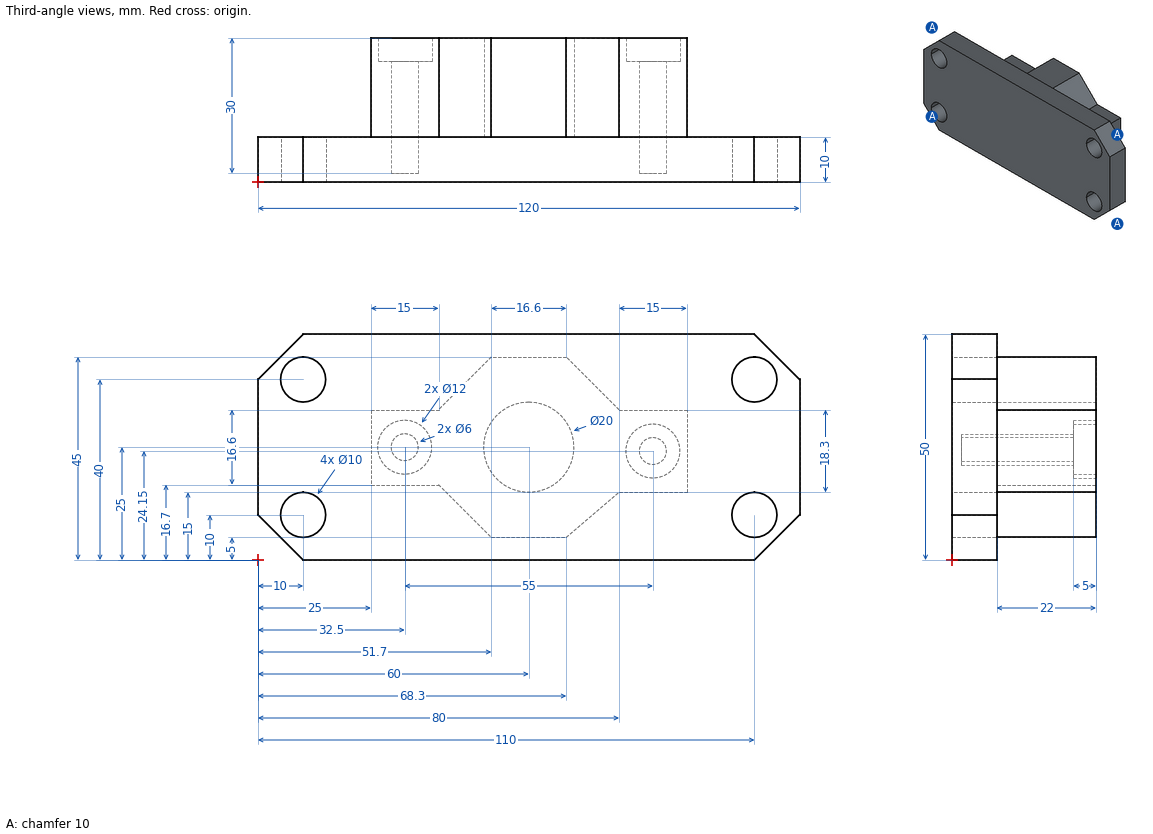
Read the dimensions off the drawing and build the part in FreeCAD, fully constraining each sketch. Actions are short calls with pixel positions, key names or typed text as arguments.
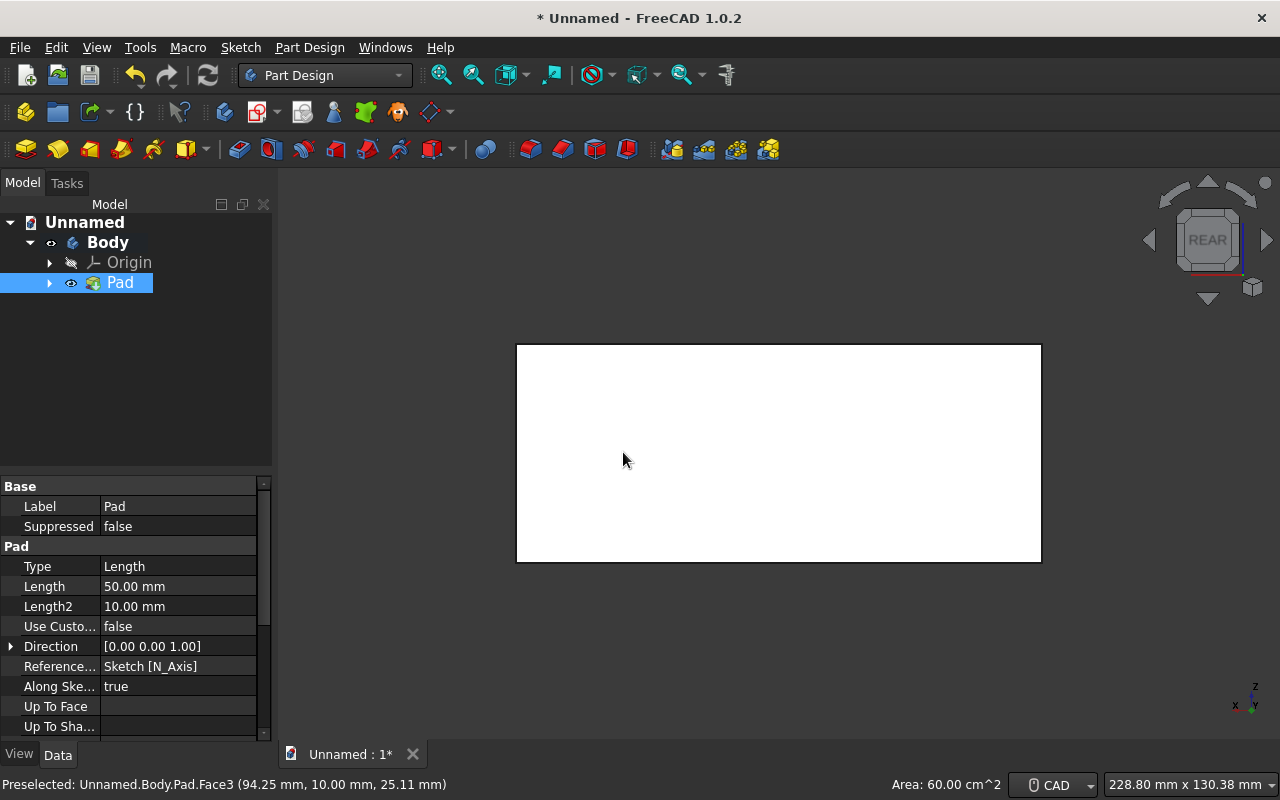
click(258, 112)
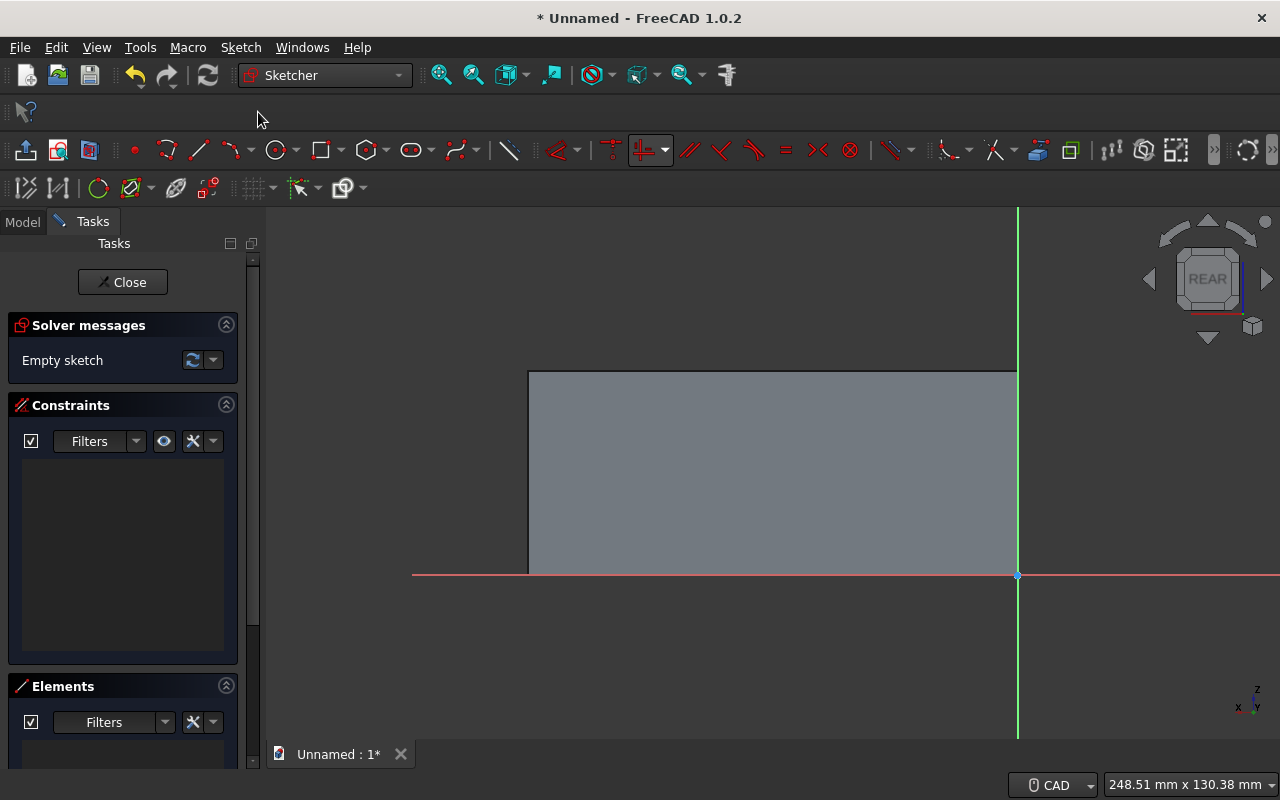
click(276, 150)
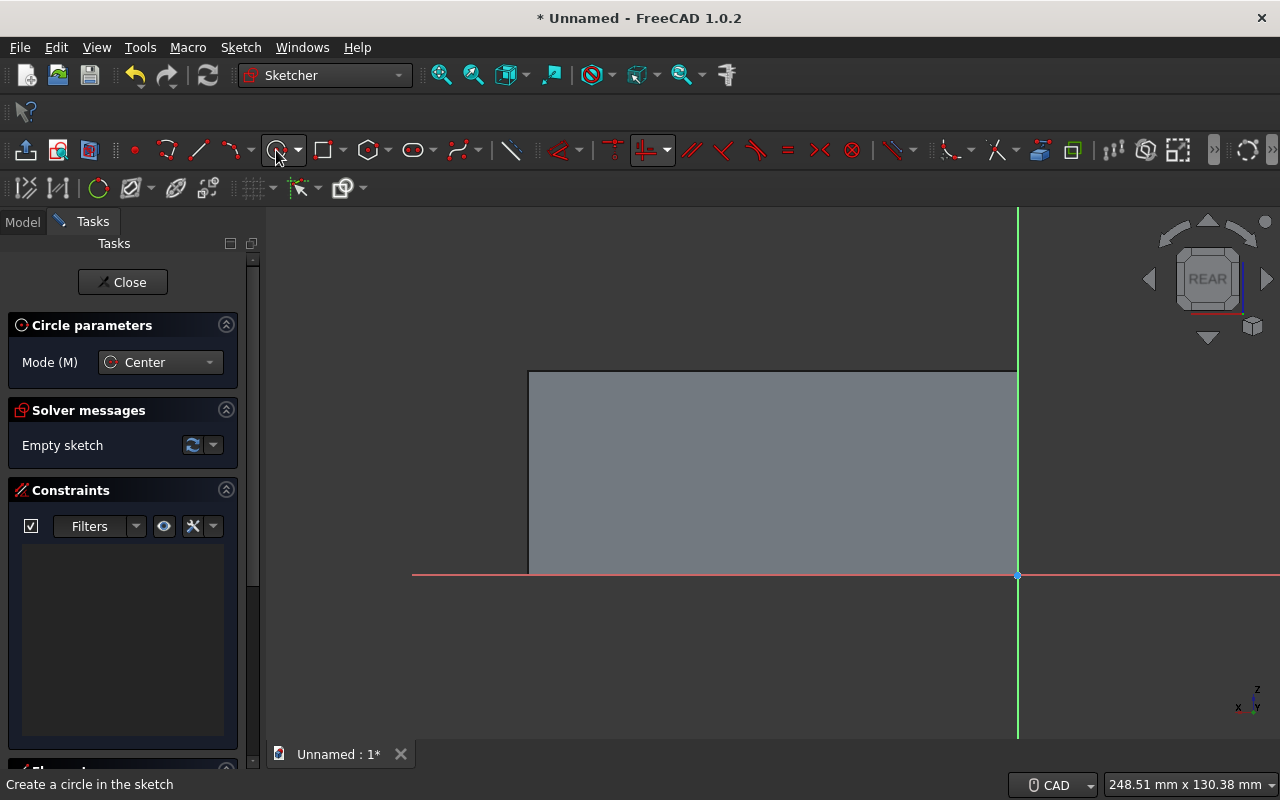
click(977, 534)
click(991, 520)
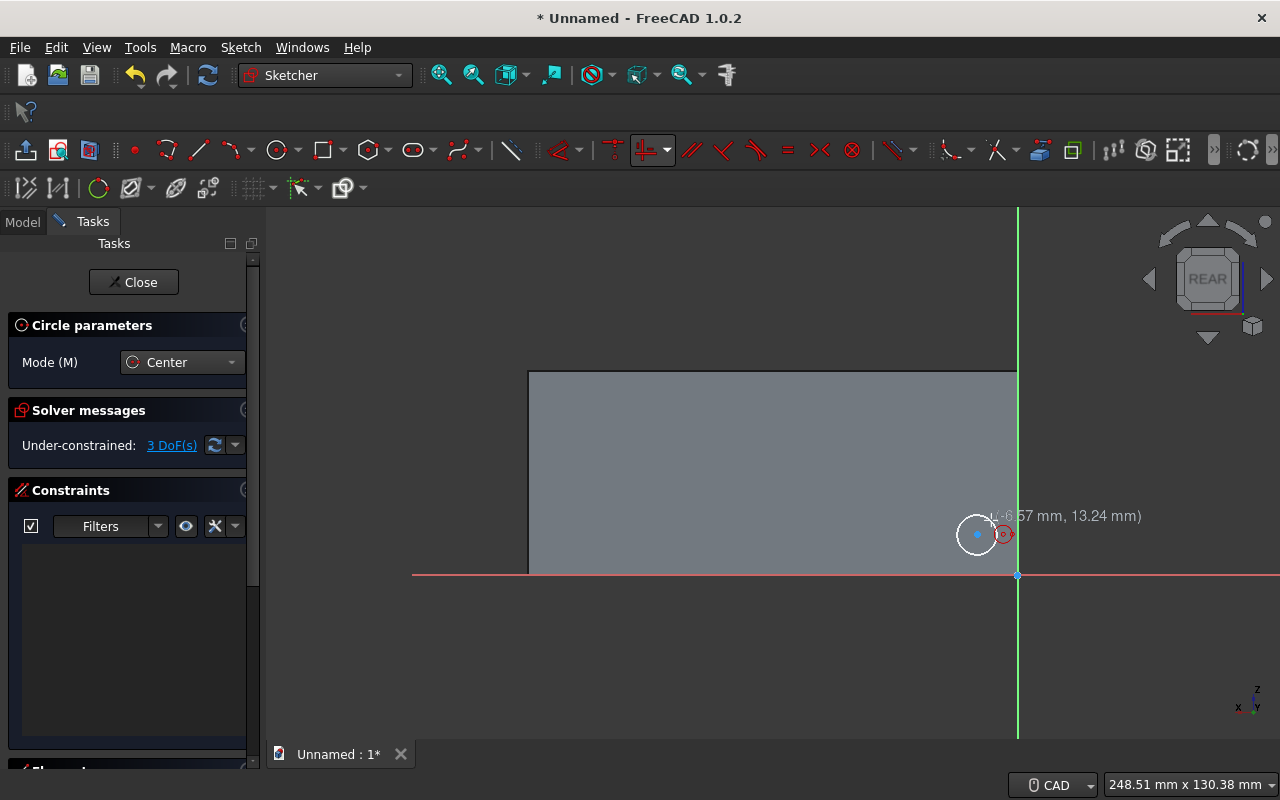
click(977, 412)
click(991, 397)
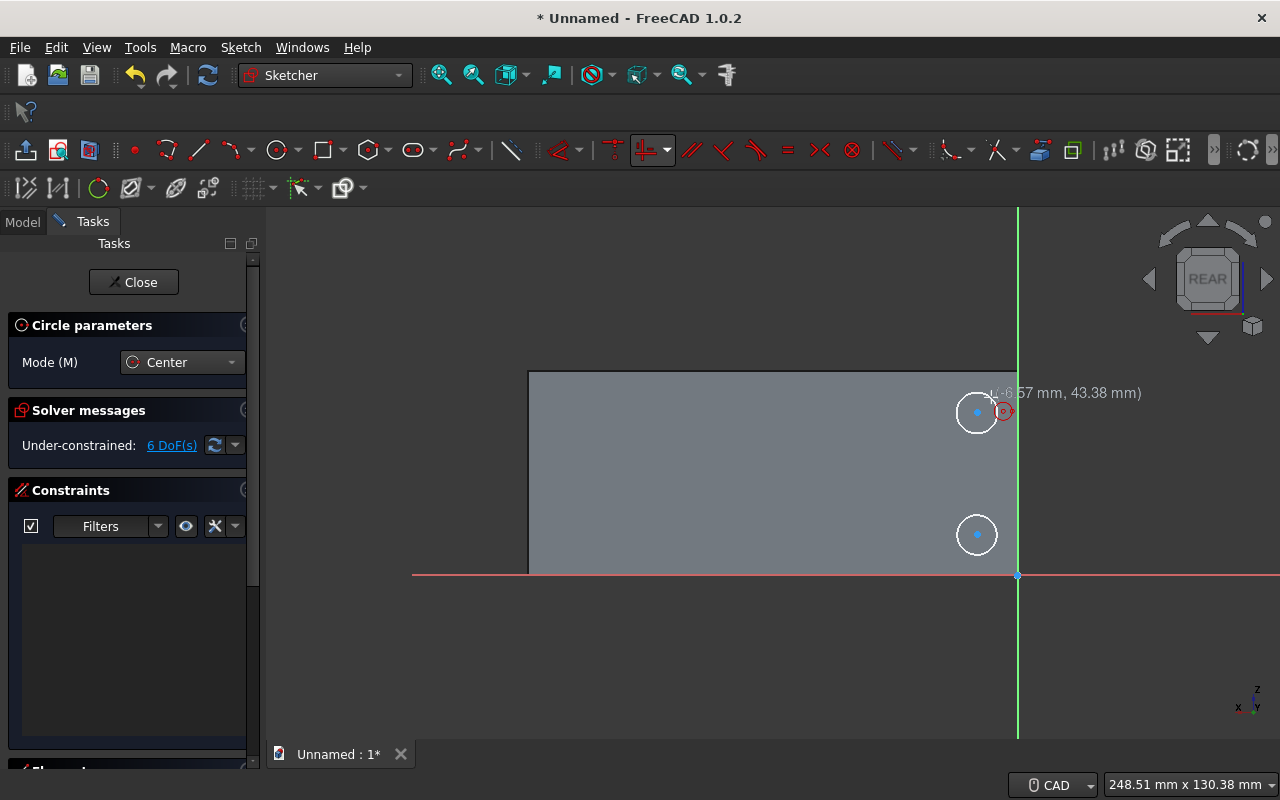
click(569, 534)
click(583, 520)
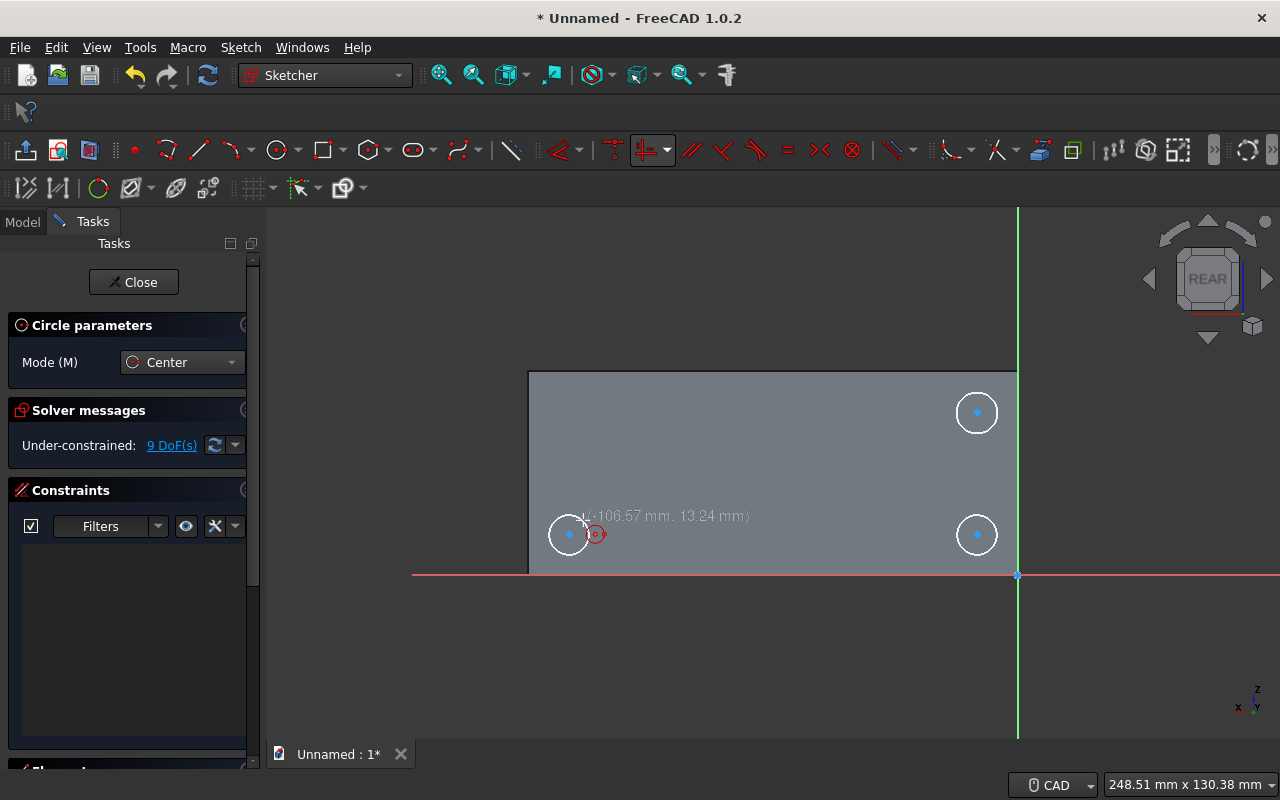
click(569, 412)
click(583, 397)
key(Escape)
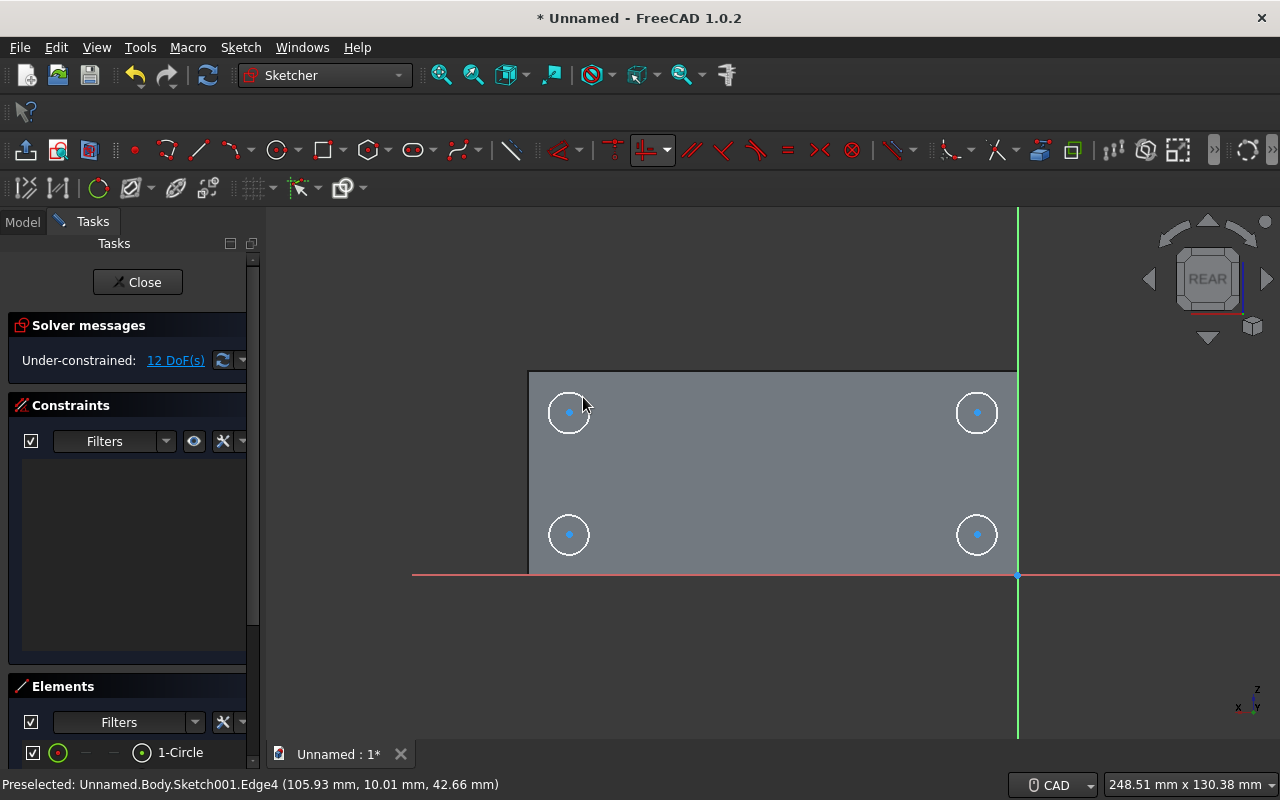
click(991, 521)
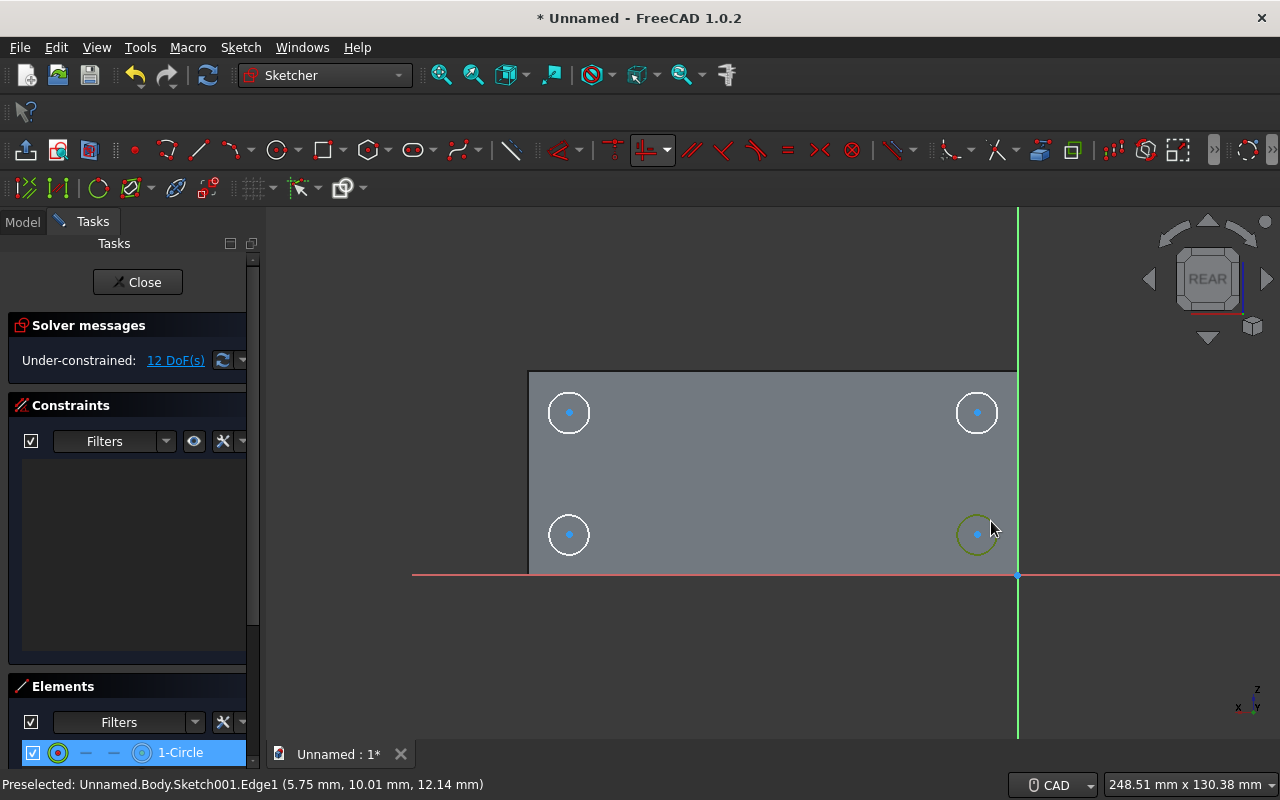
click(991, 398)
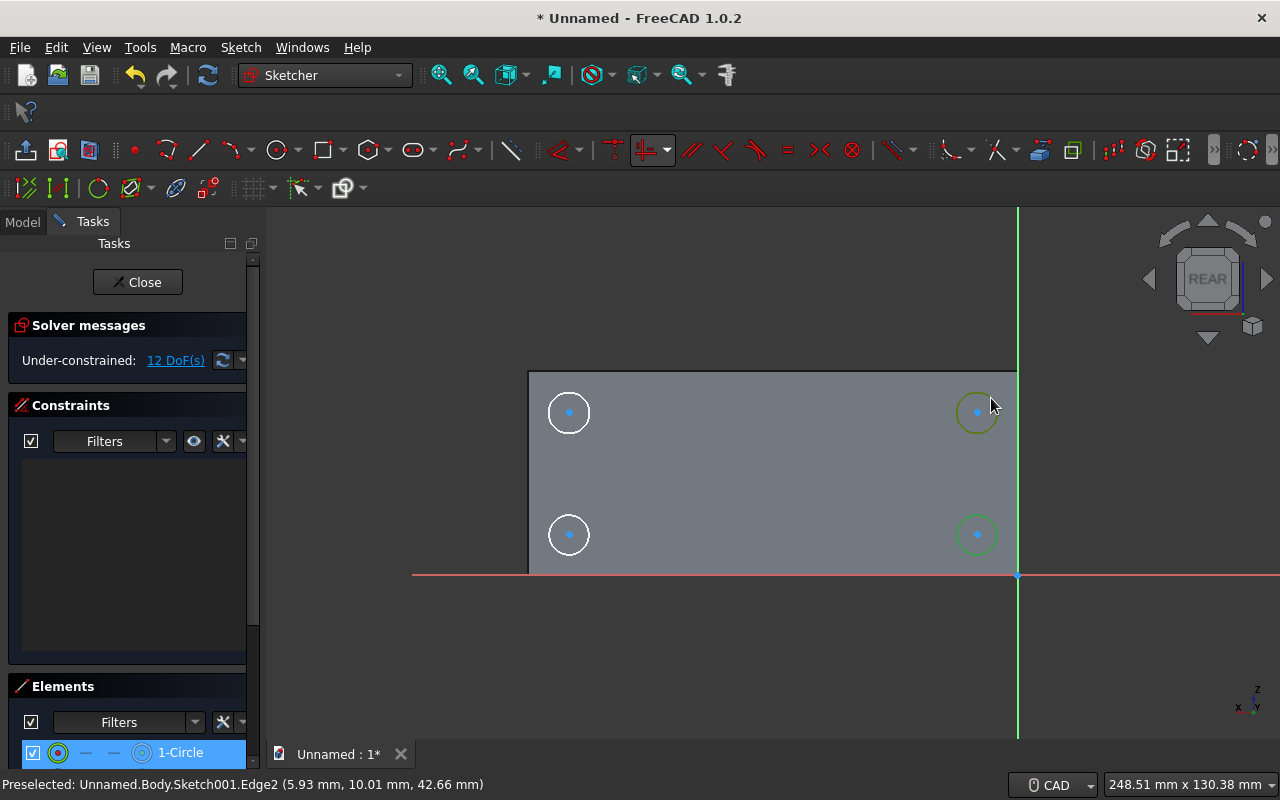
click(583, 521)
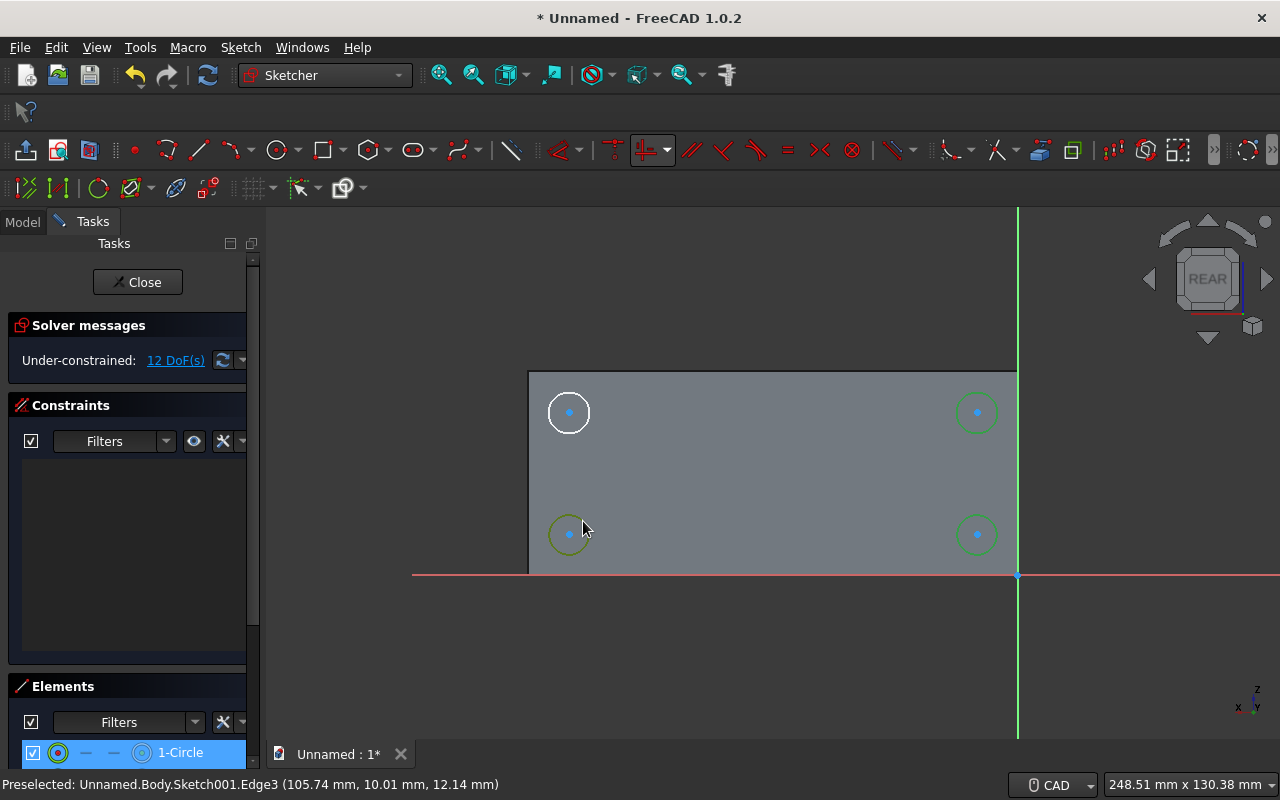
click(583, 398)